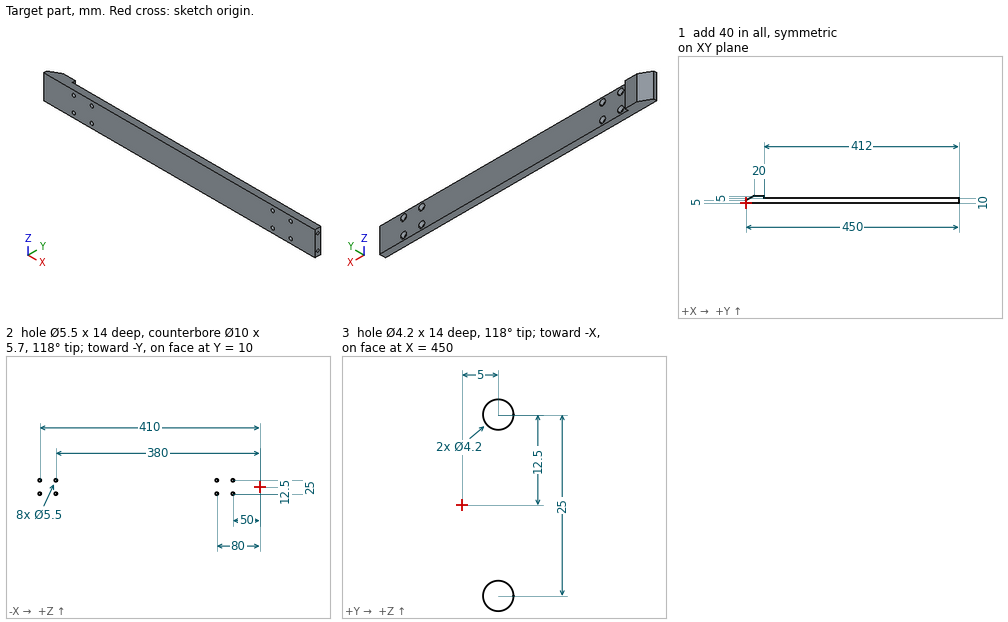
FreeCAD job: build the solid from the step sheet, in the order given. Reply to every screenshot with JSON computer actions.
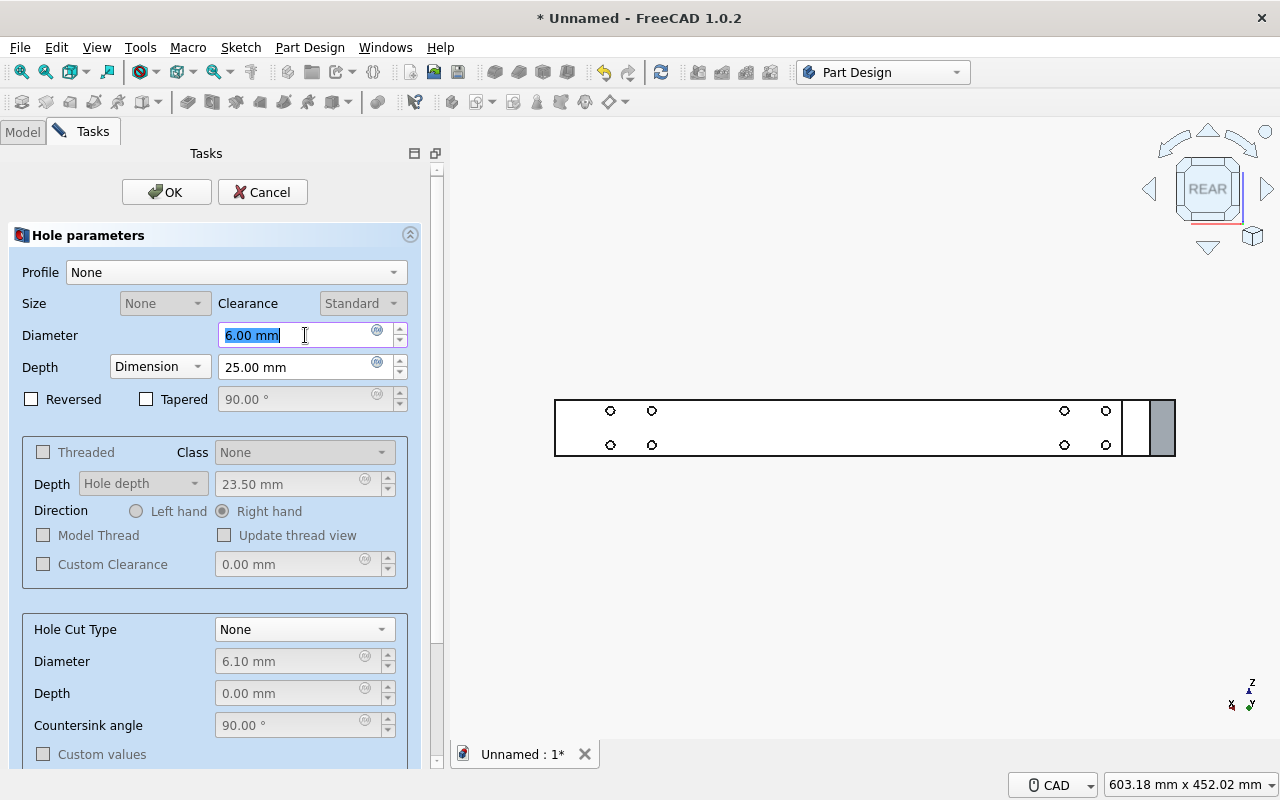
{"action": "type", "text": "5.5"}
{"action": "key", "text": "Tab"}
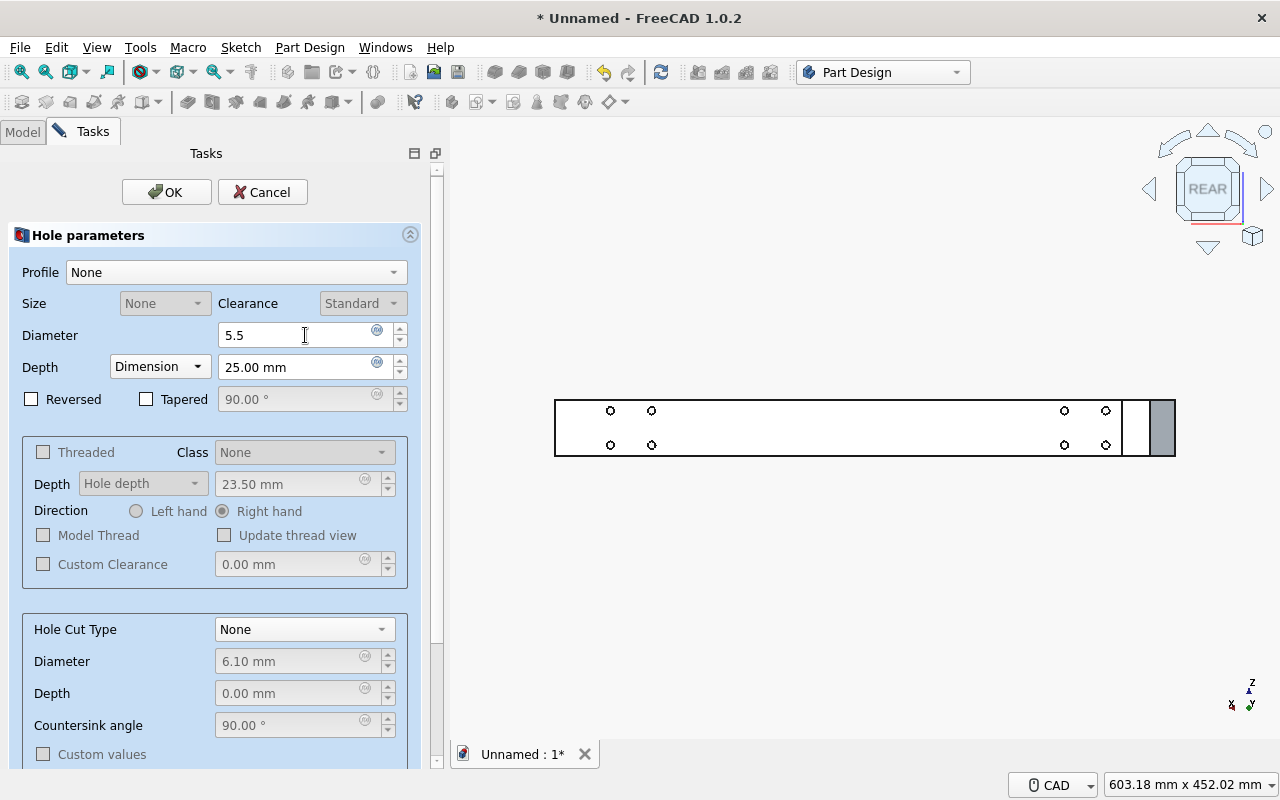
{"action": "triple_click", "coordinate": [305, 367]}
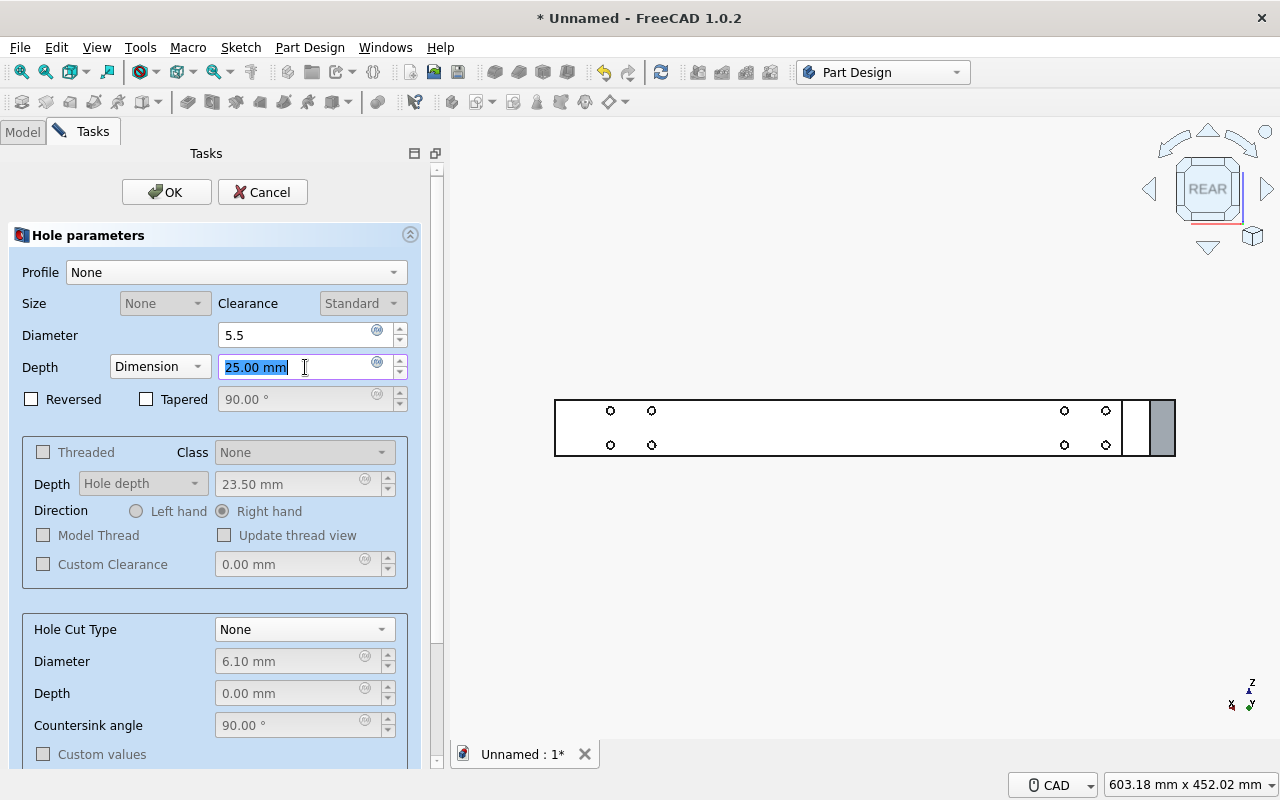
{"action": "type", "text": "14"}
{"action": "key", "text": "Tab"}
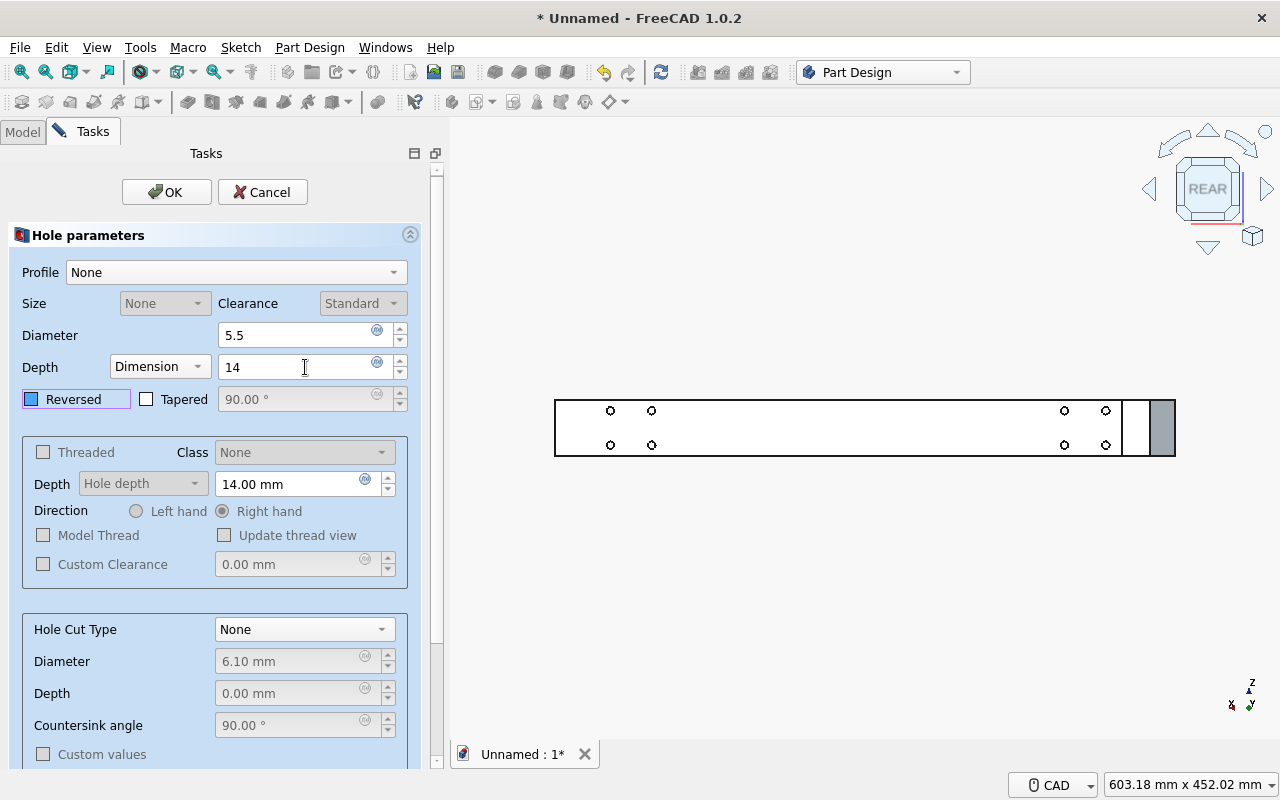
{"action": "left_click", "coordinate": [306, 630]}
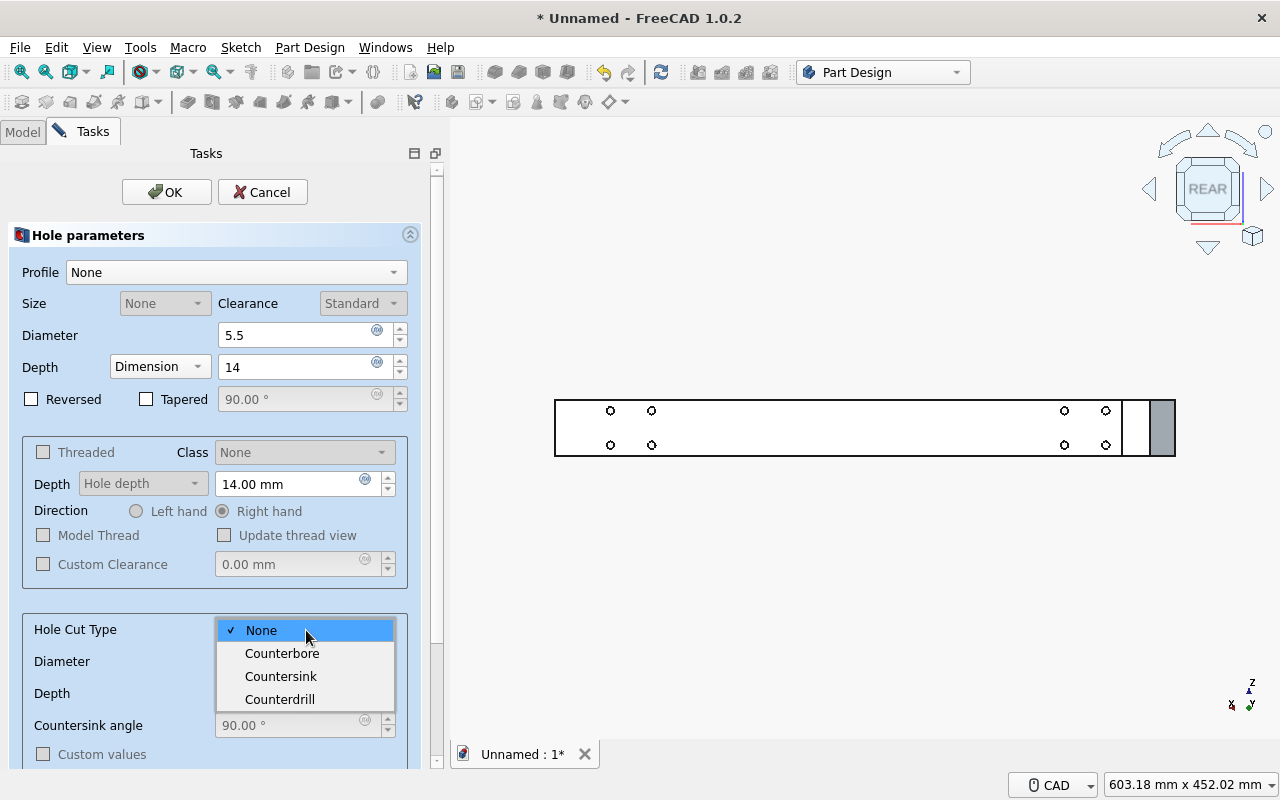
{"action": "left_click", "coordinate": [304, 654]}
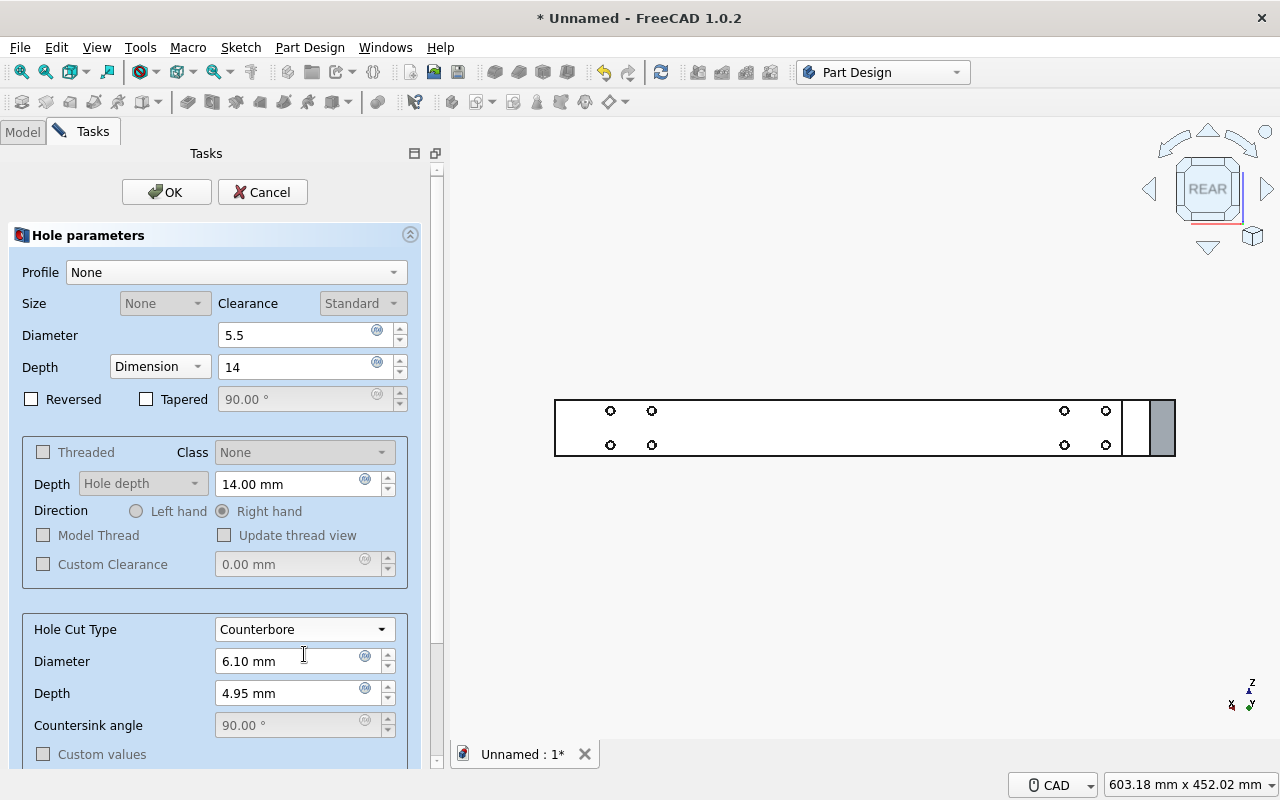
{"action": "triple_click", "coordinate": [298, 661]}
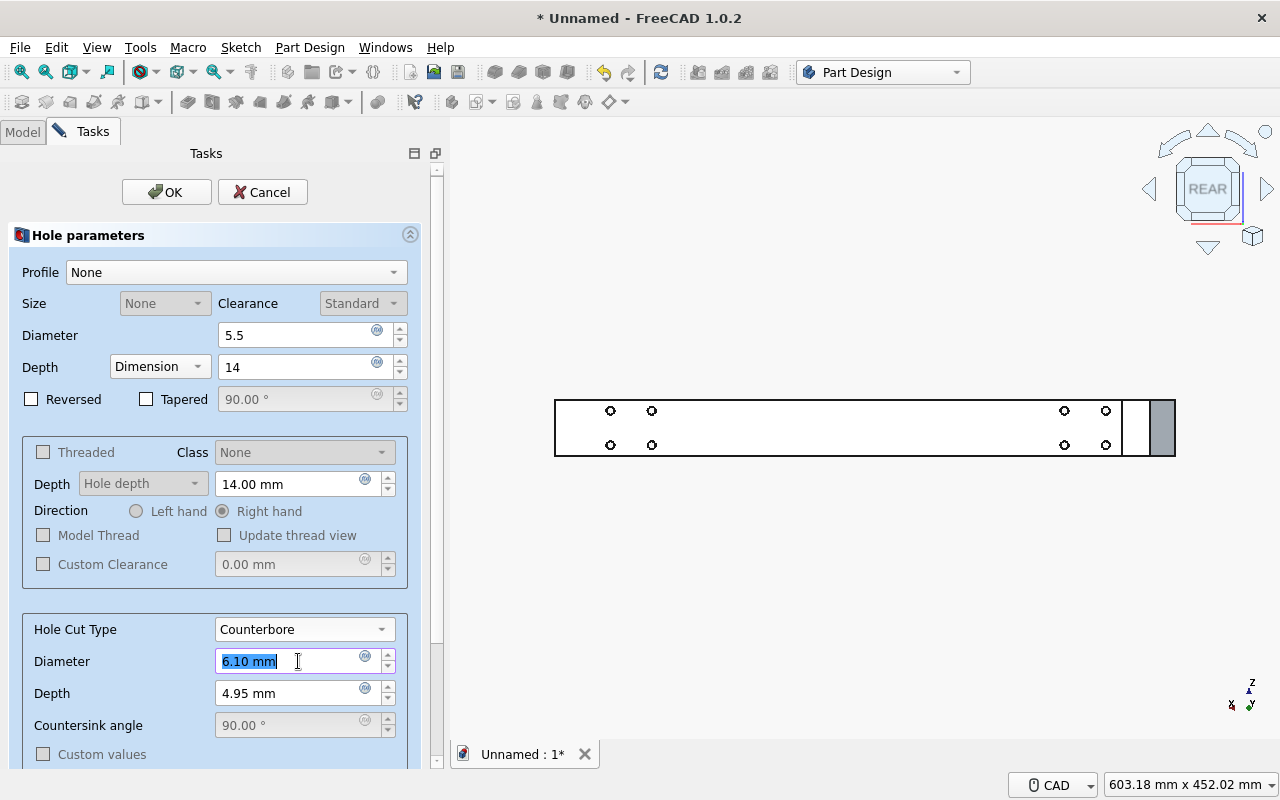
{"action": "type", "text": "10"}
{"action": "key", "text": "Tab"}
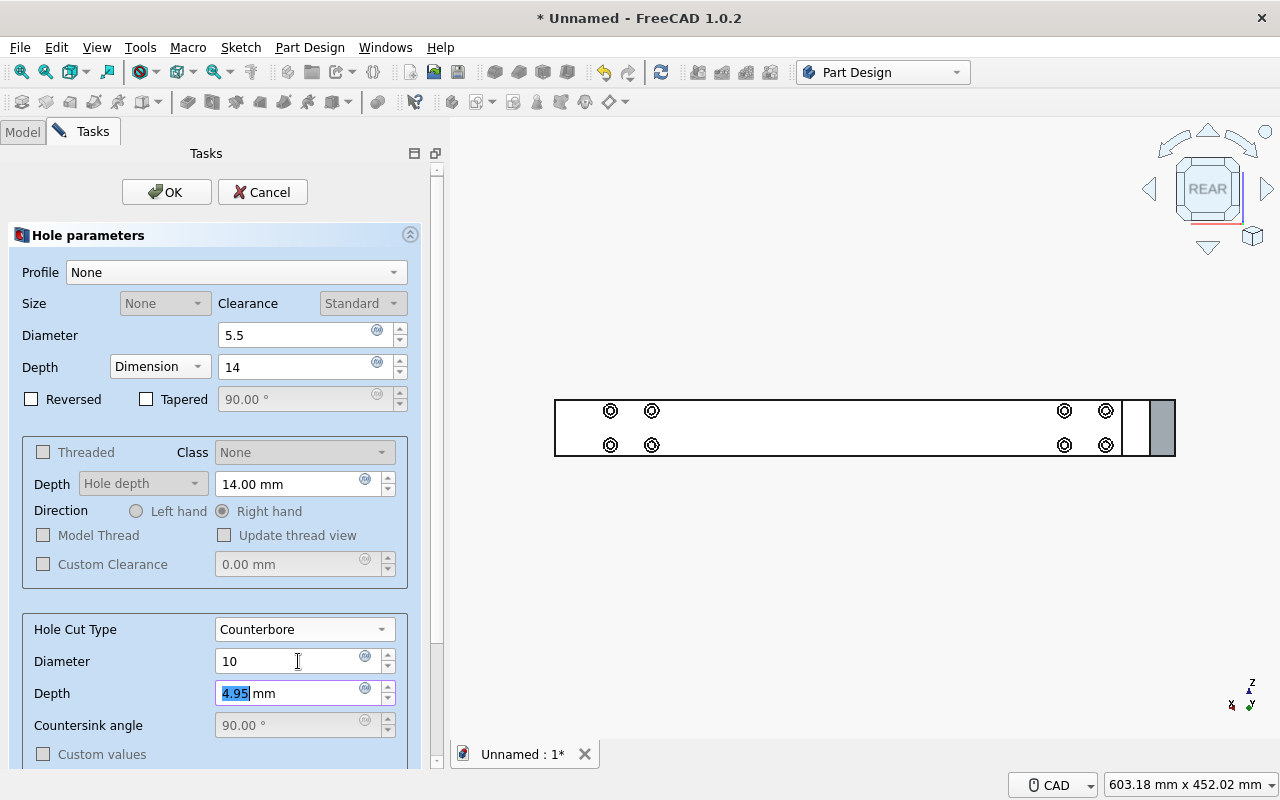
{"action": "type", "text": "5.7"}
{"action": "key", "text": "Tab"}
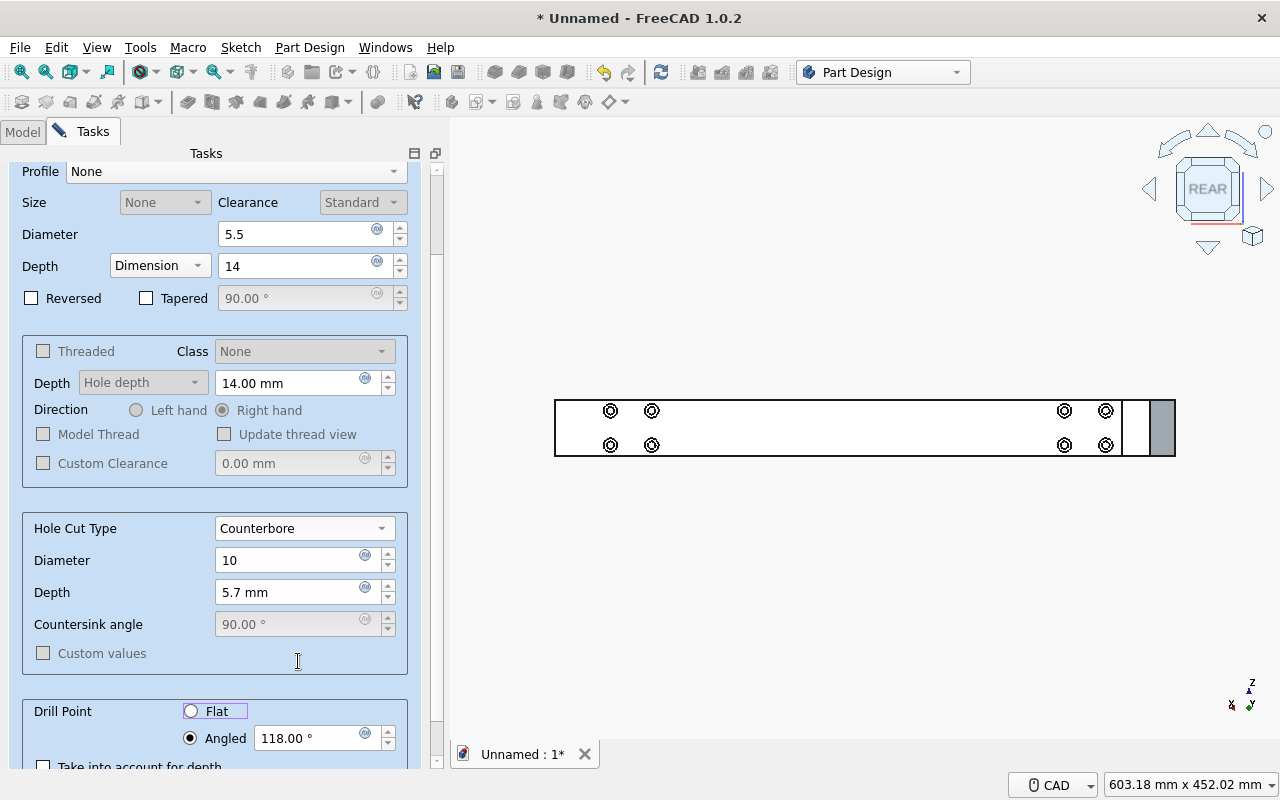
{"action": "scroll", "coordinate": [437, 466], "scroll_direction": "up", "scroll_amount": 3}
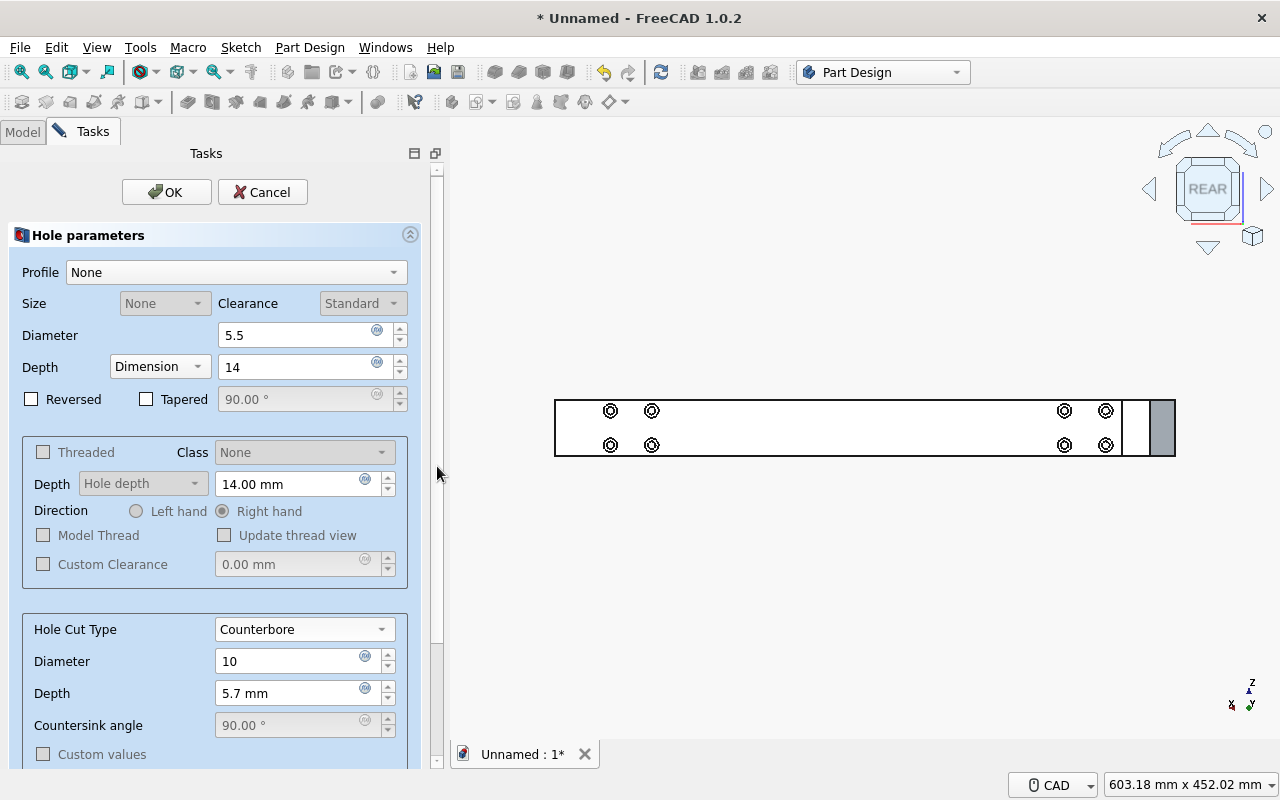
{"action": "left_click", "coordinate": [167, 192]}